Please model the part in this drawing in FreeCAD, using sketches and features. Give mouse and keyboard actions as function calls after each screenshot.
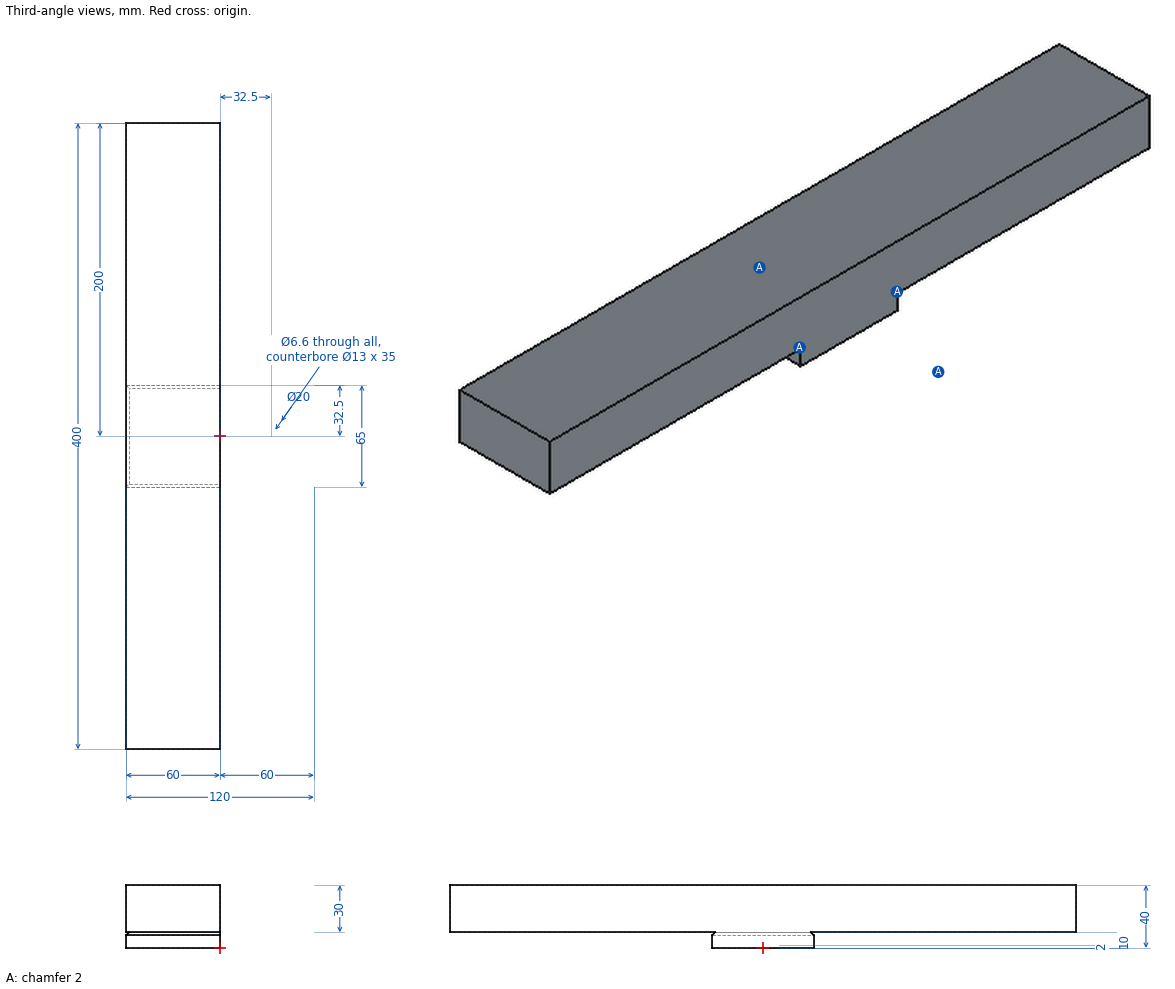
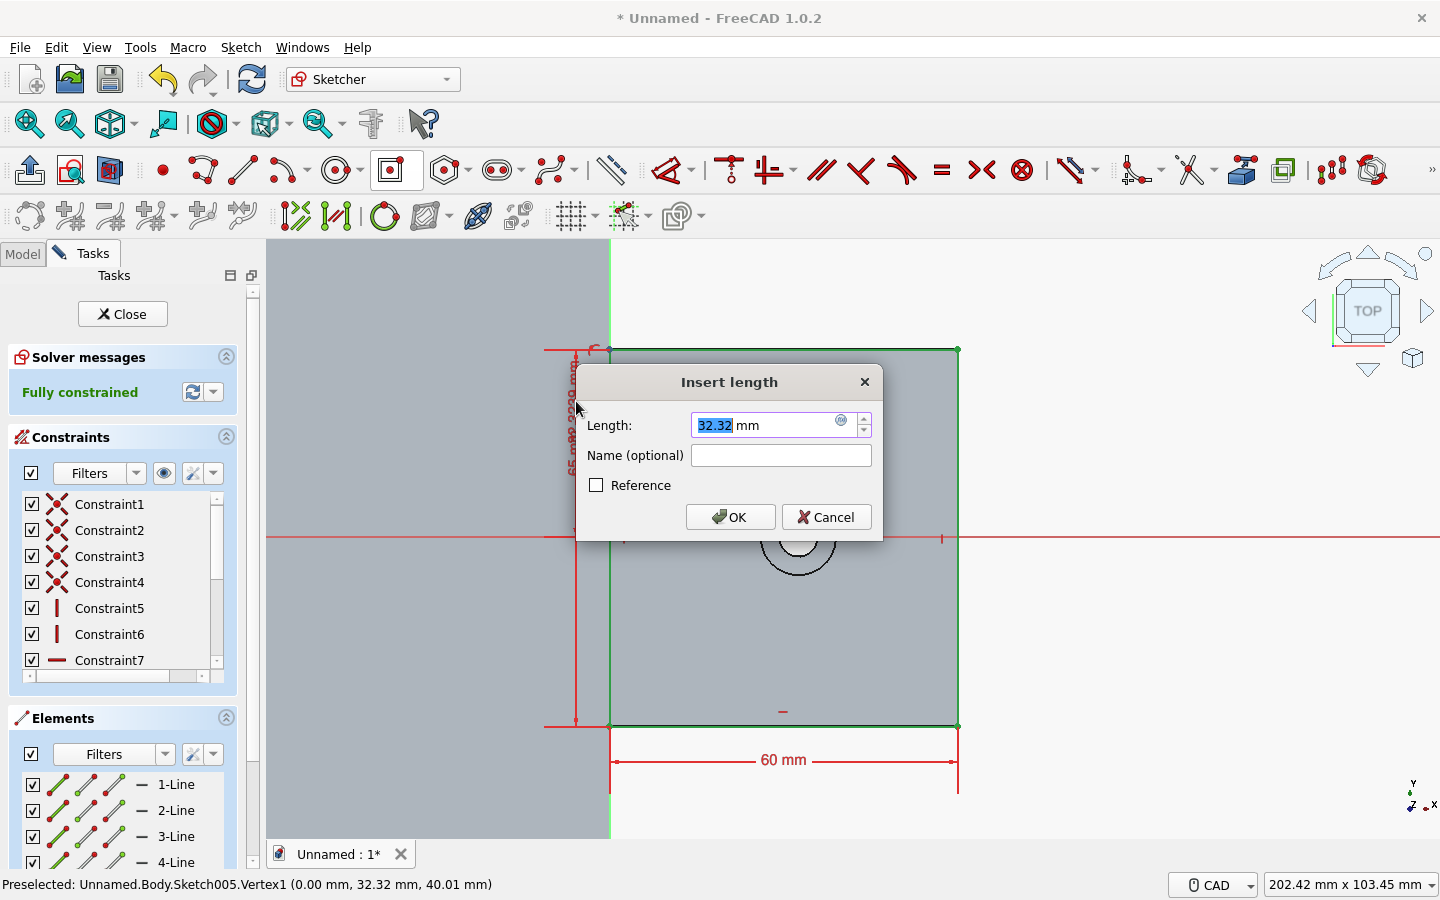
text(32.5)
key(Return)
key(Escape)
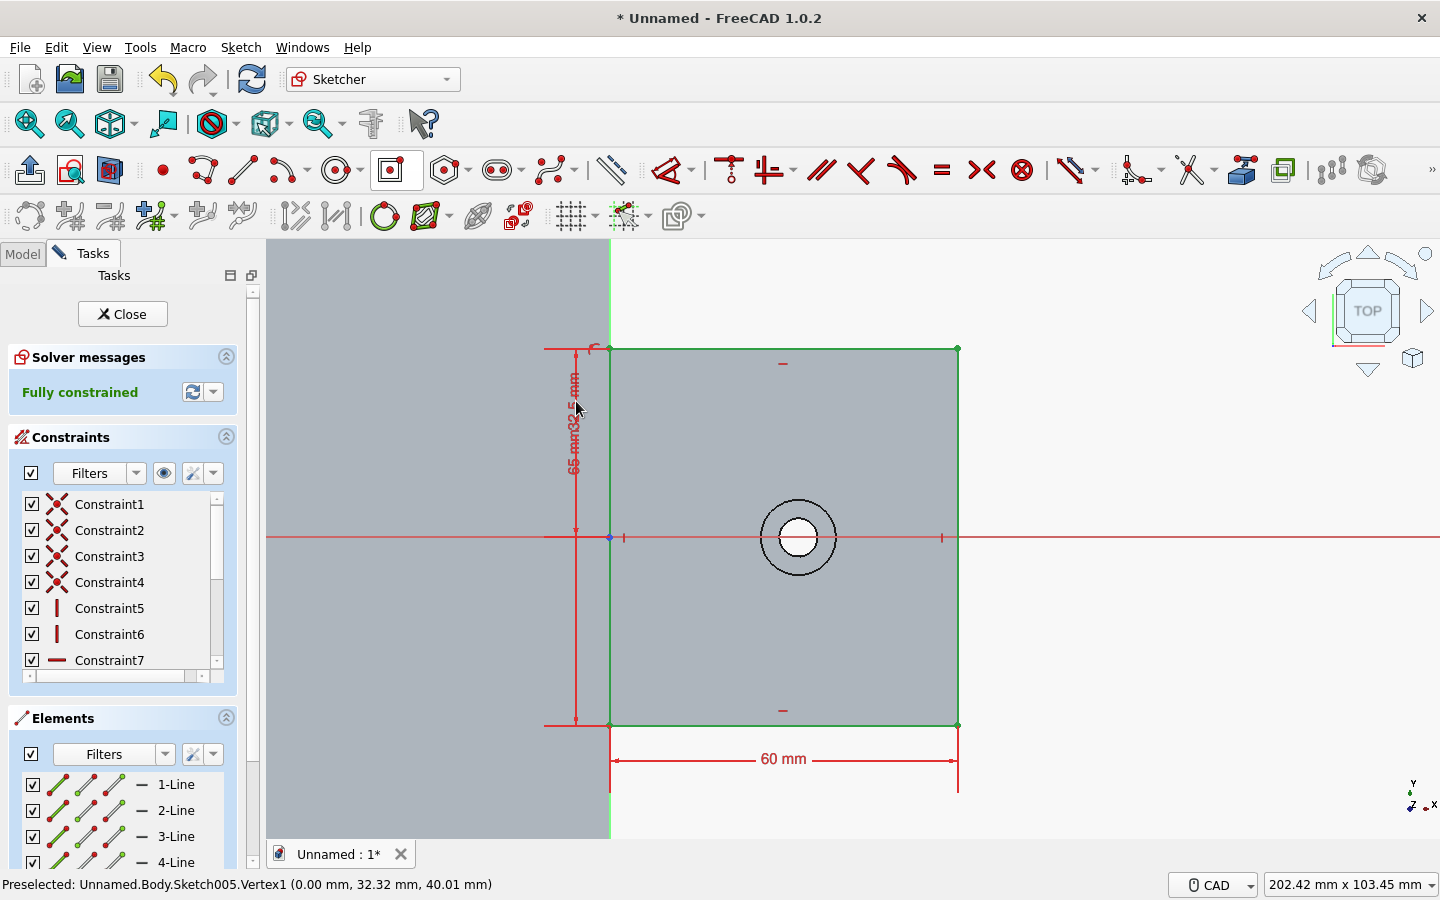
click(123, 314)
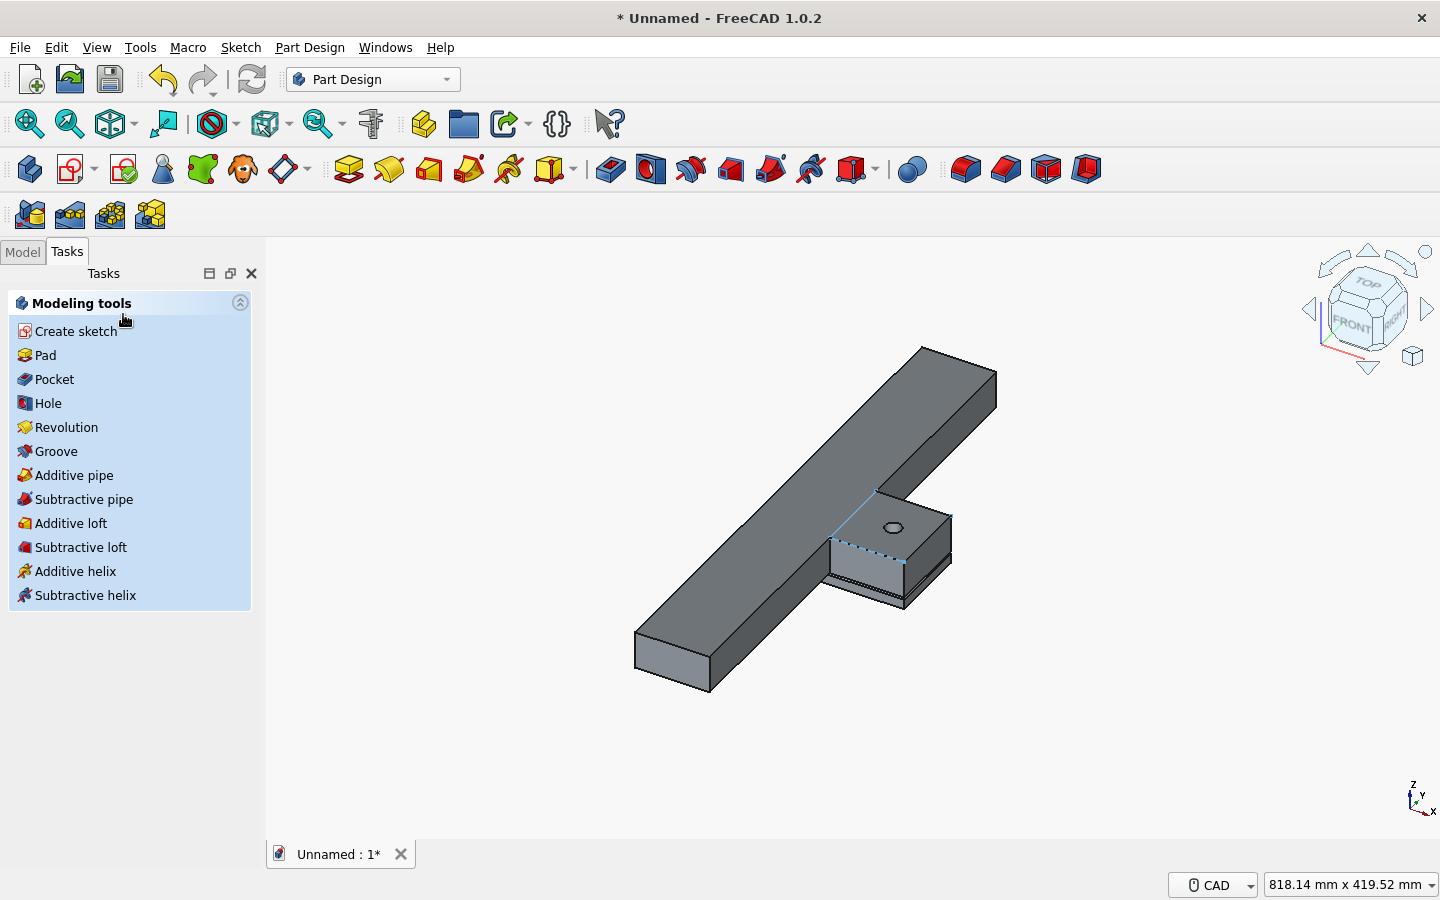
click(612, 170)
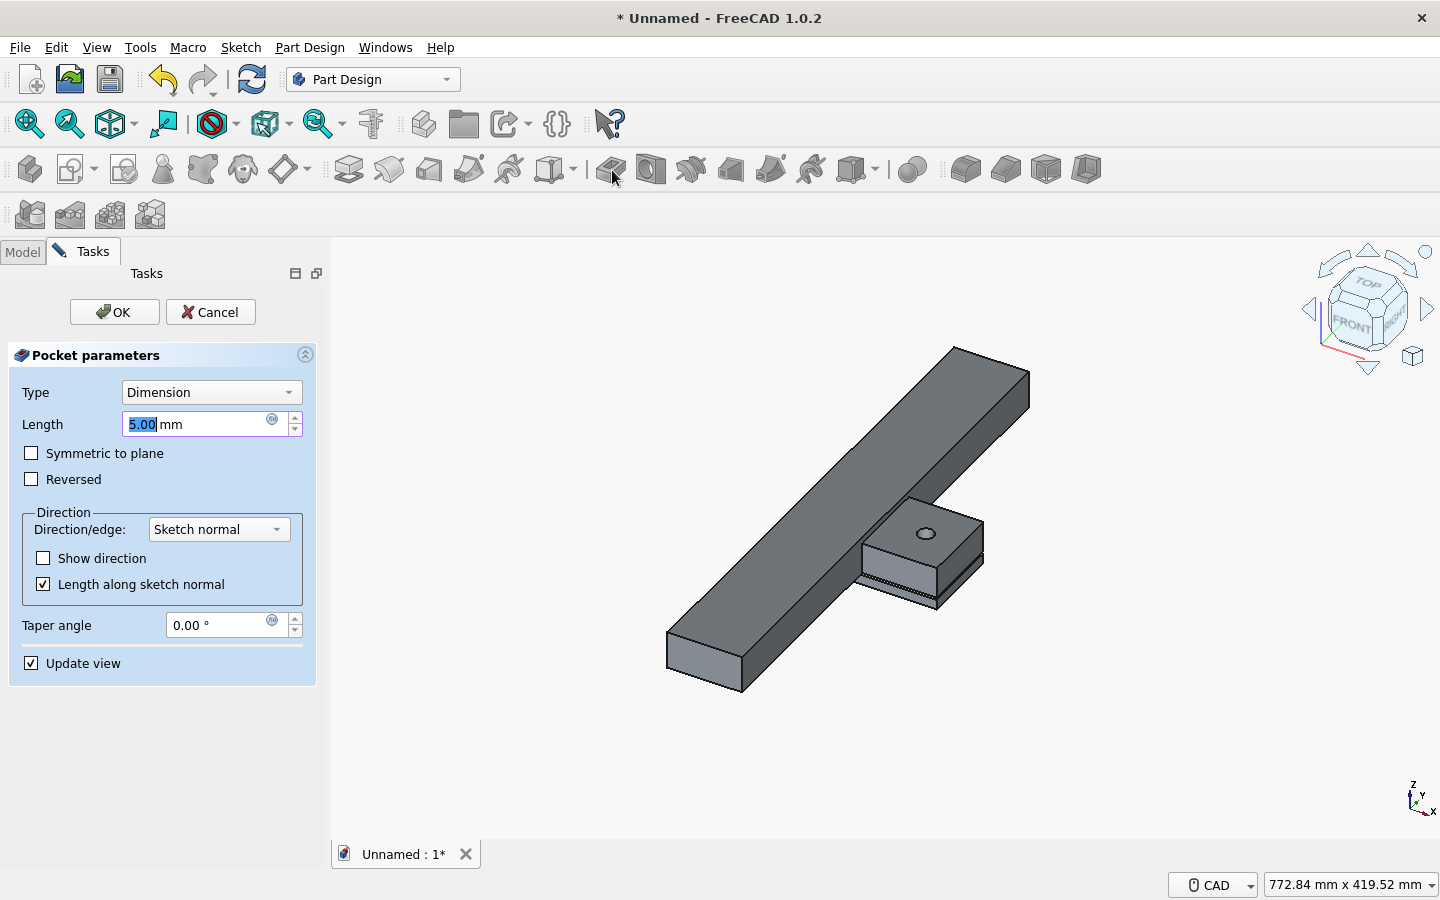
text(40)
key(Tab)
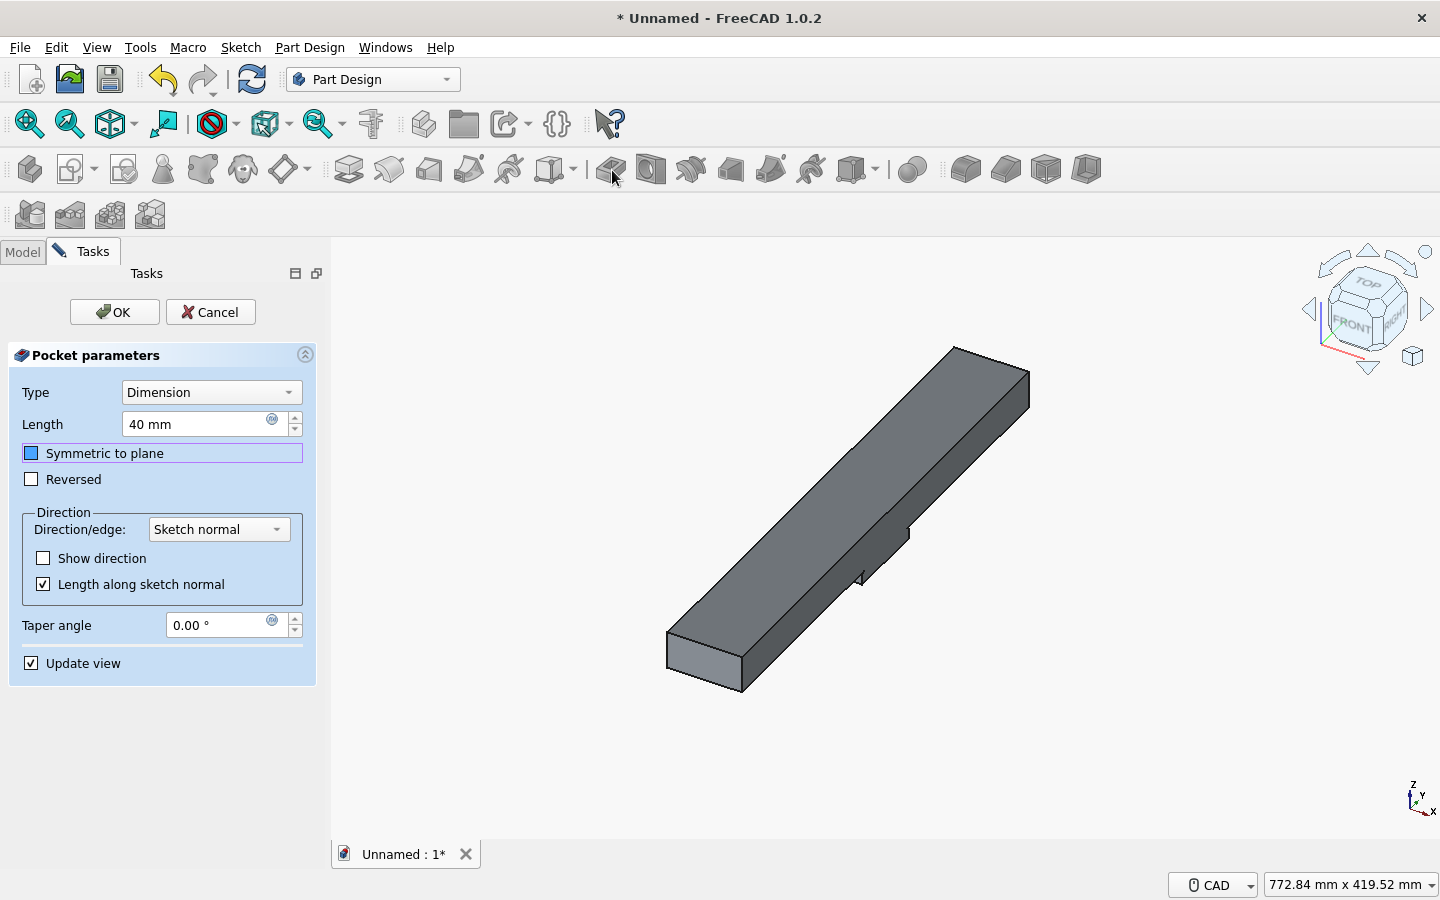
click(115, 312)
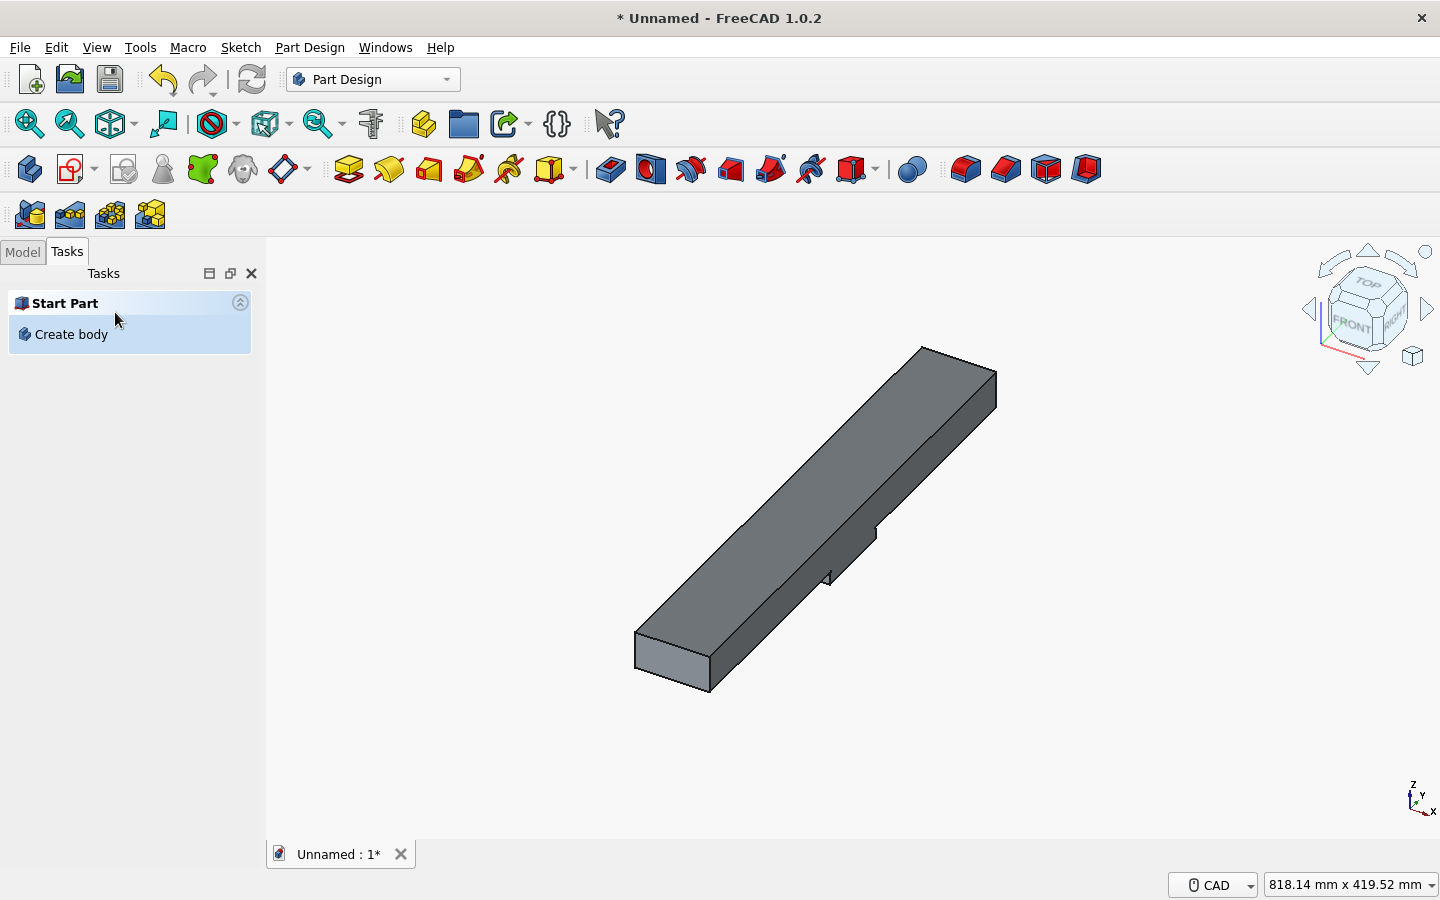
key(0)